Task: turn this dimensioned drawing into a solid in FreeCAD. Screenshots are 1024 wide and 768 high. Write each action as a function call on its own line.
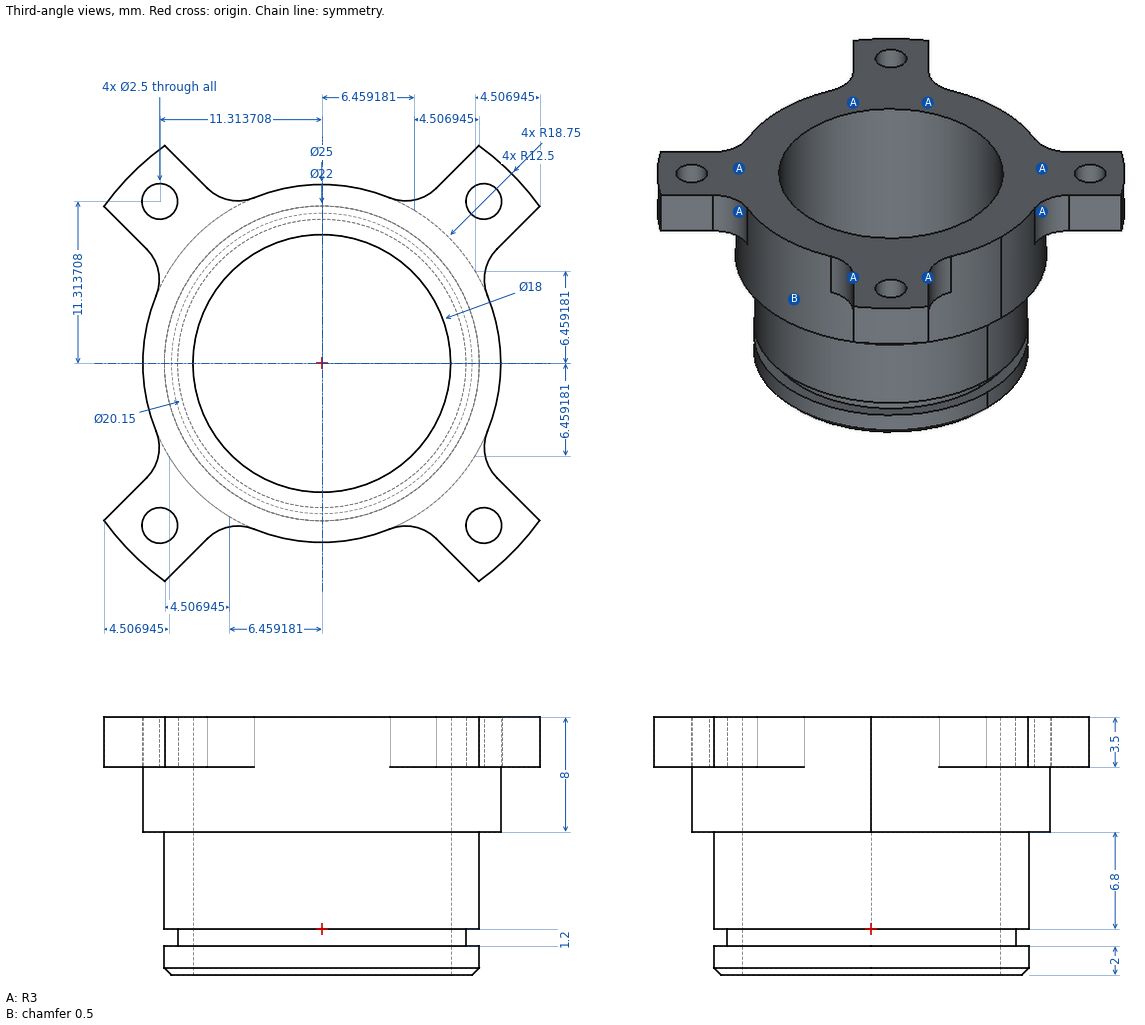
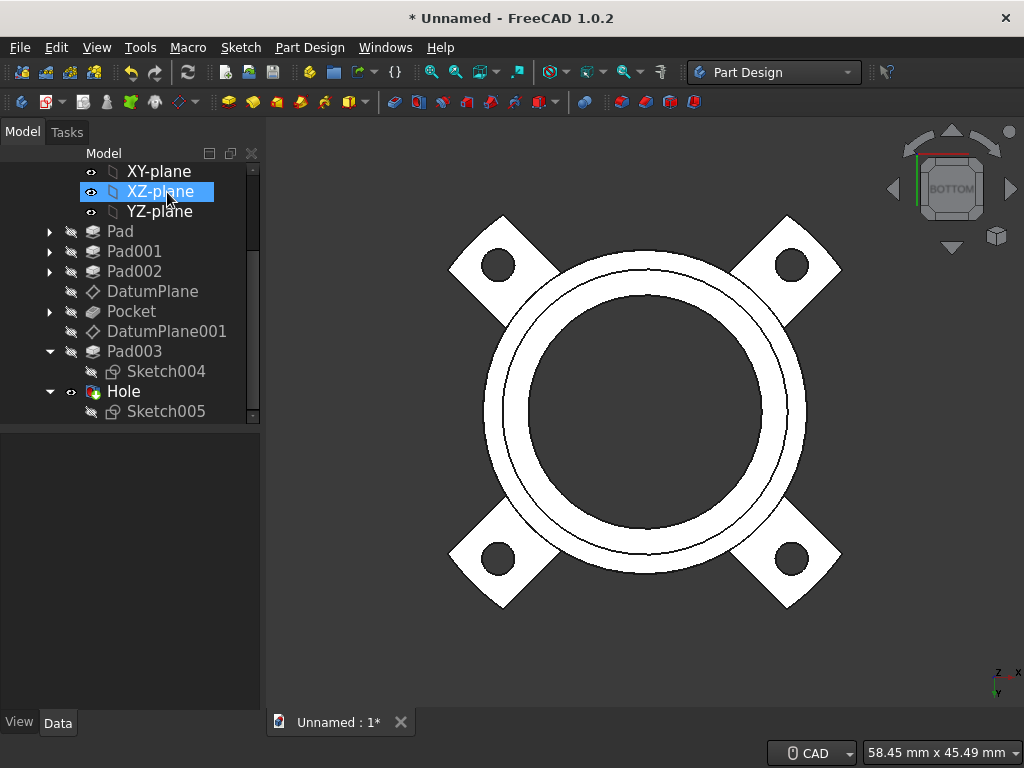
key(4)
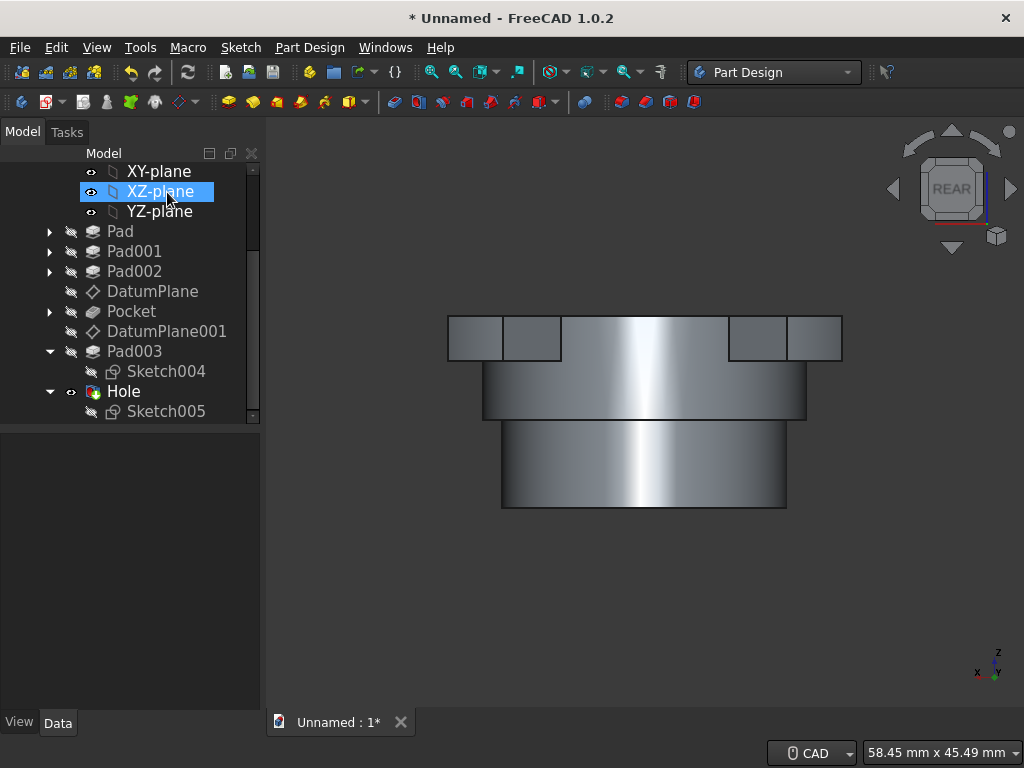
key(6)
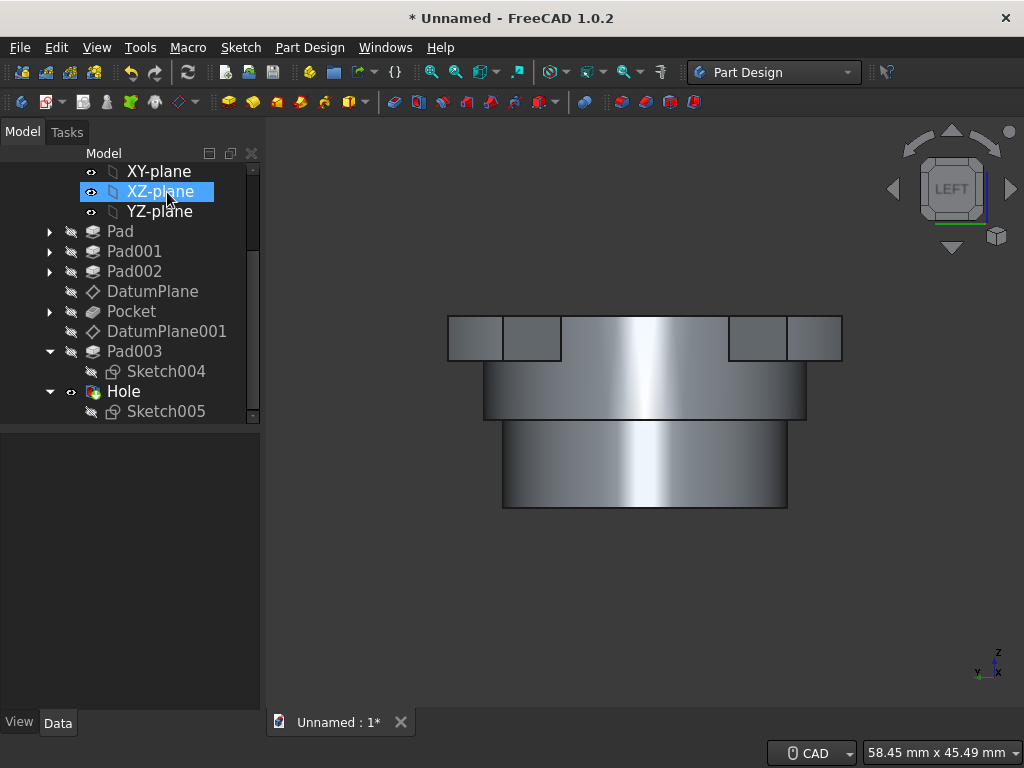
key(v)
key(3)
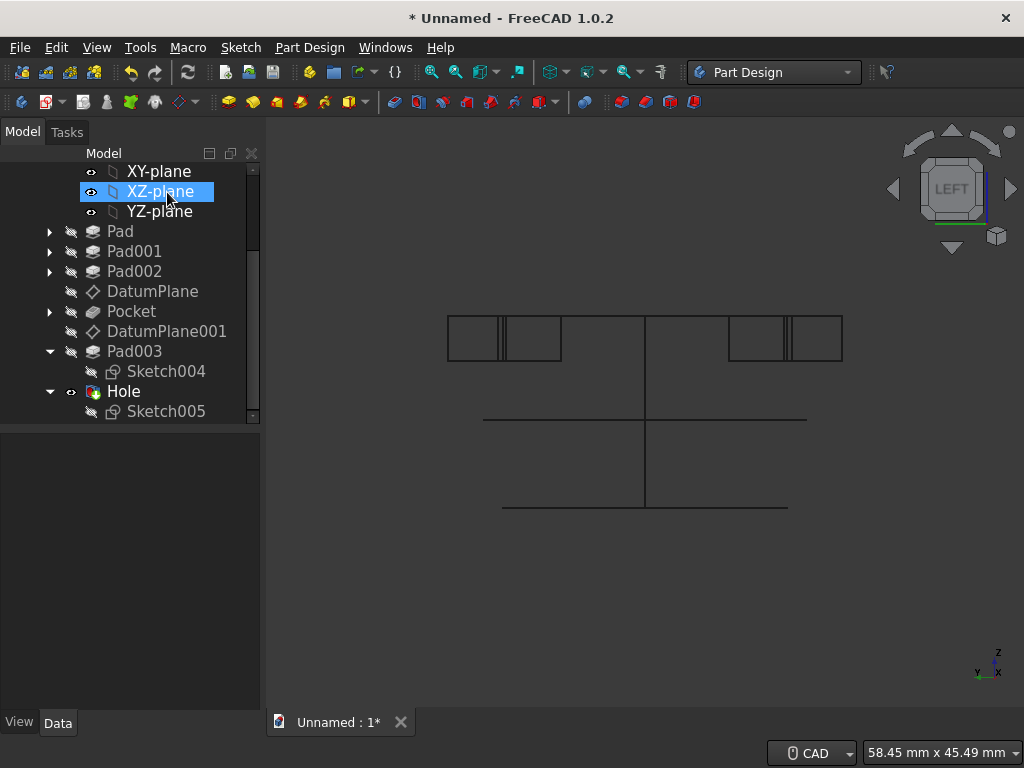
key(0)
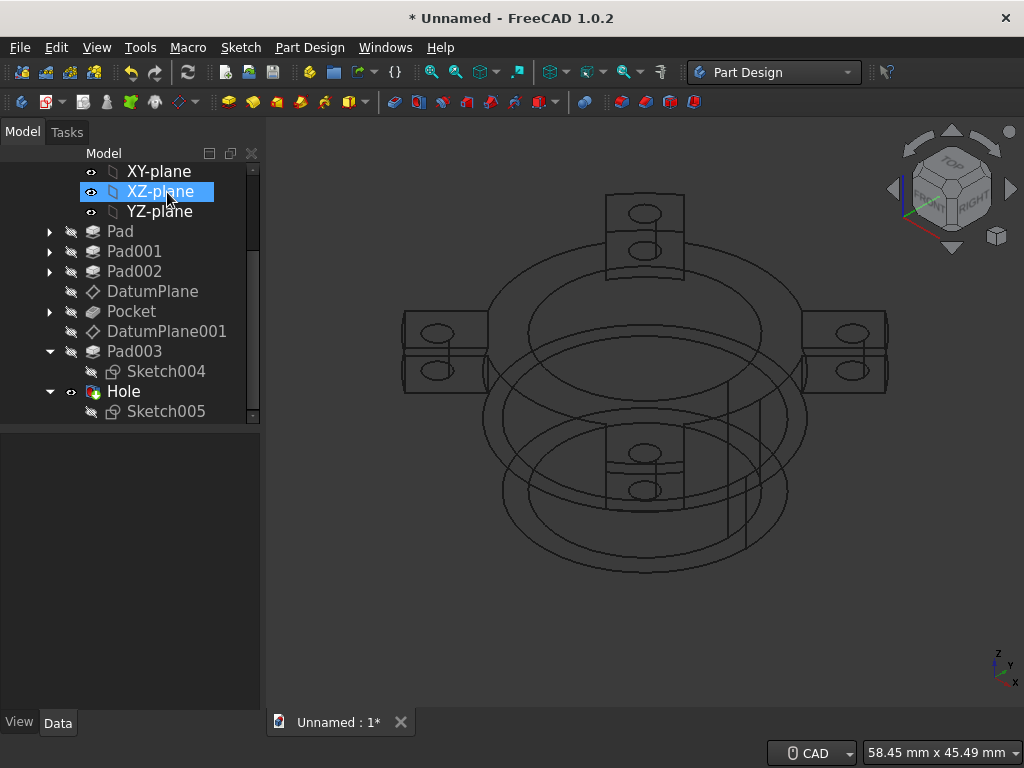
click(802, 374)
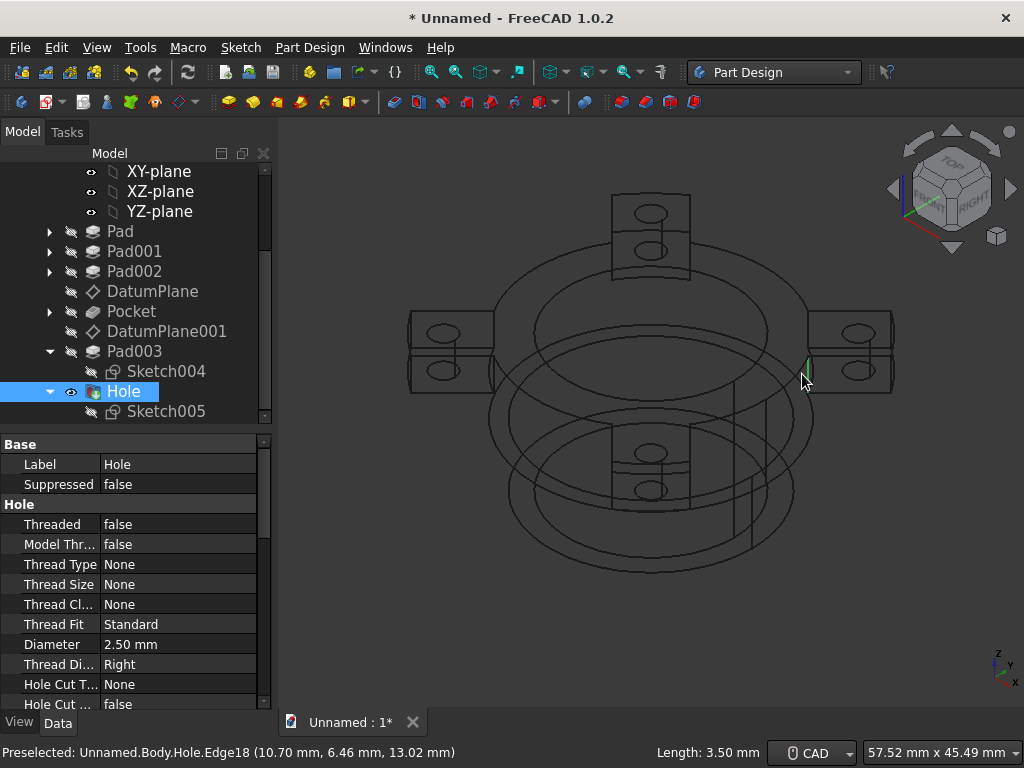
click(808, 329, ctrl)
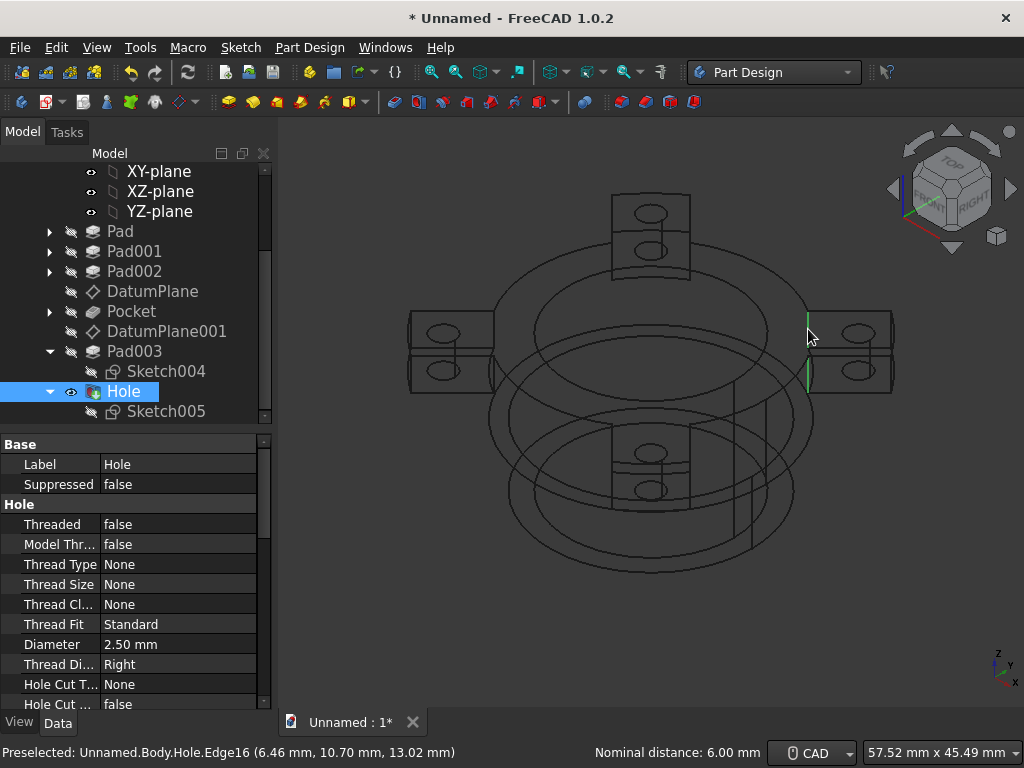
click(494, 329, ctrl)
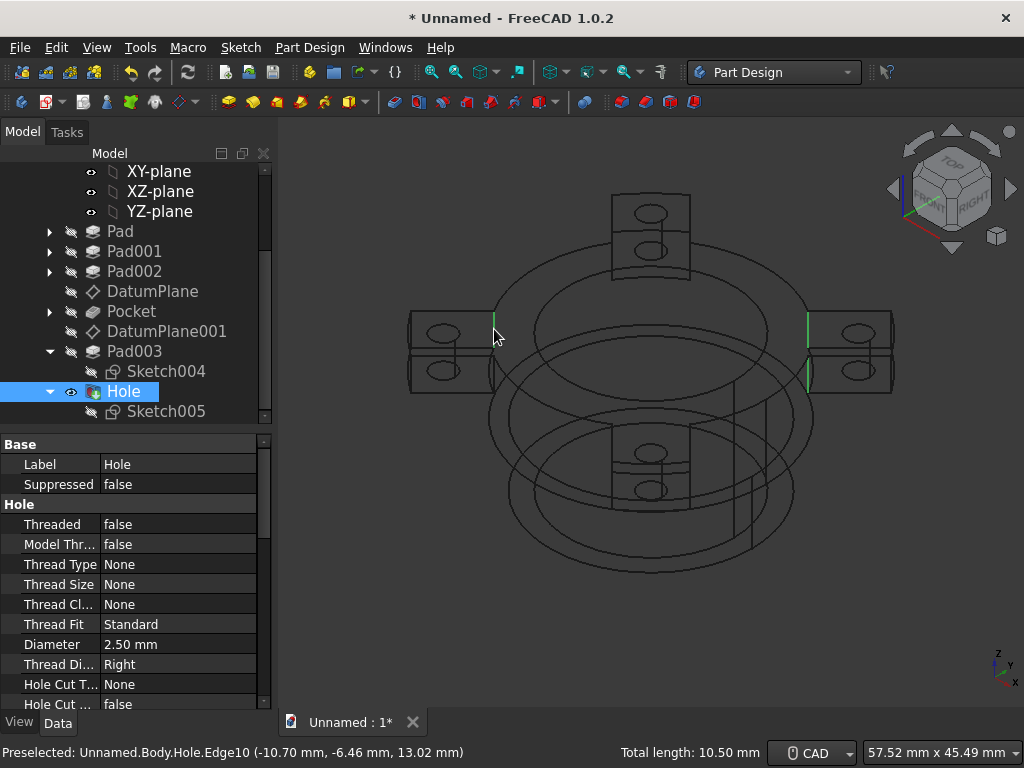
click(494, 374, ctrl)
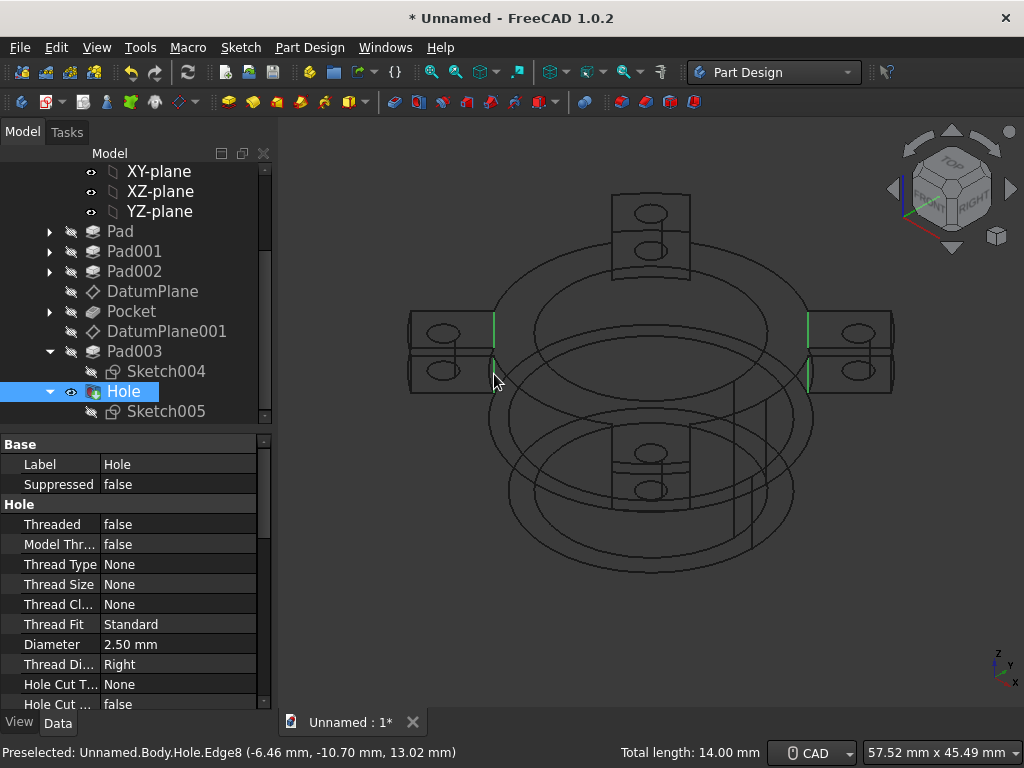
click(690, 260, ctrl)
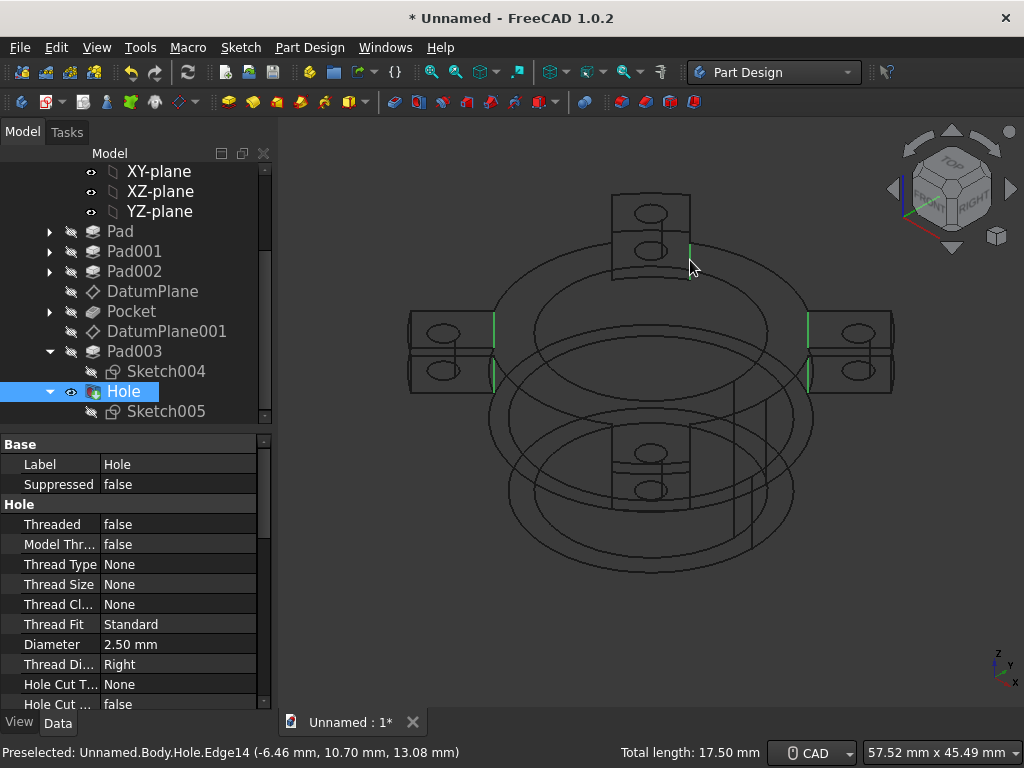
click(612, 260, ctrl)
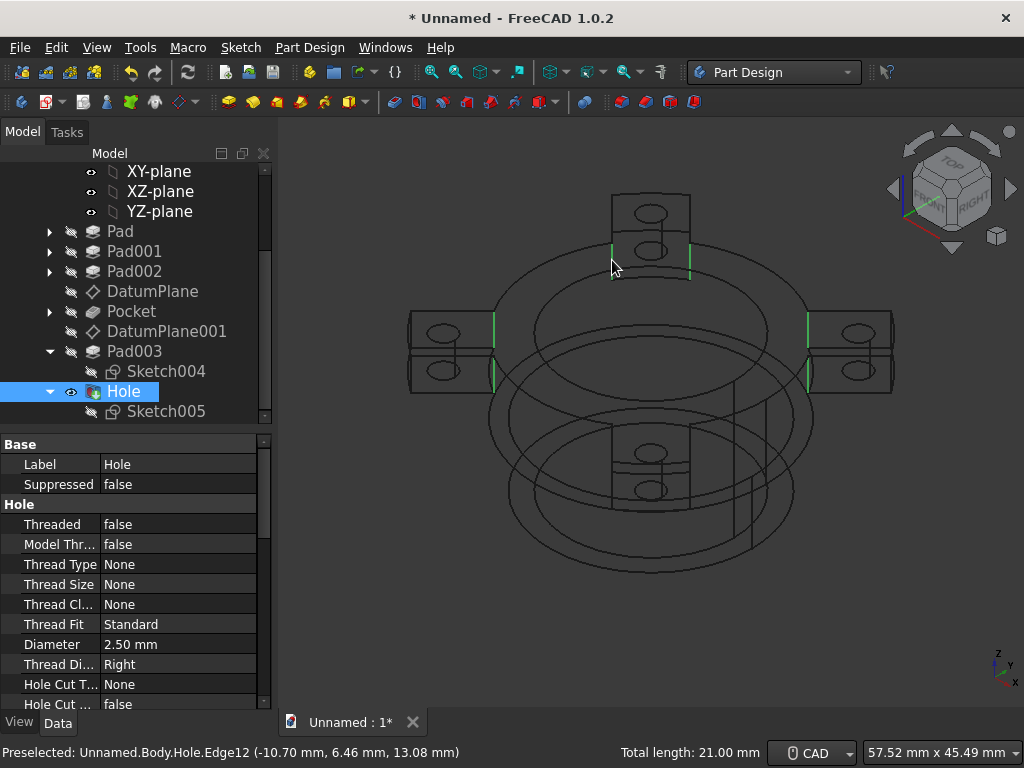
key(2)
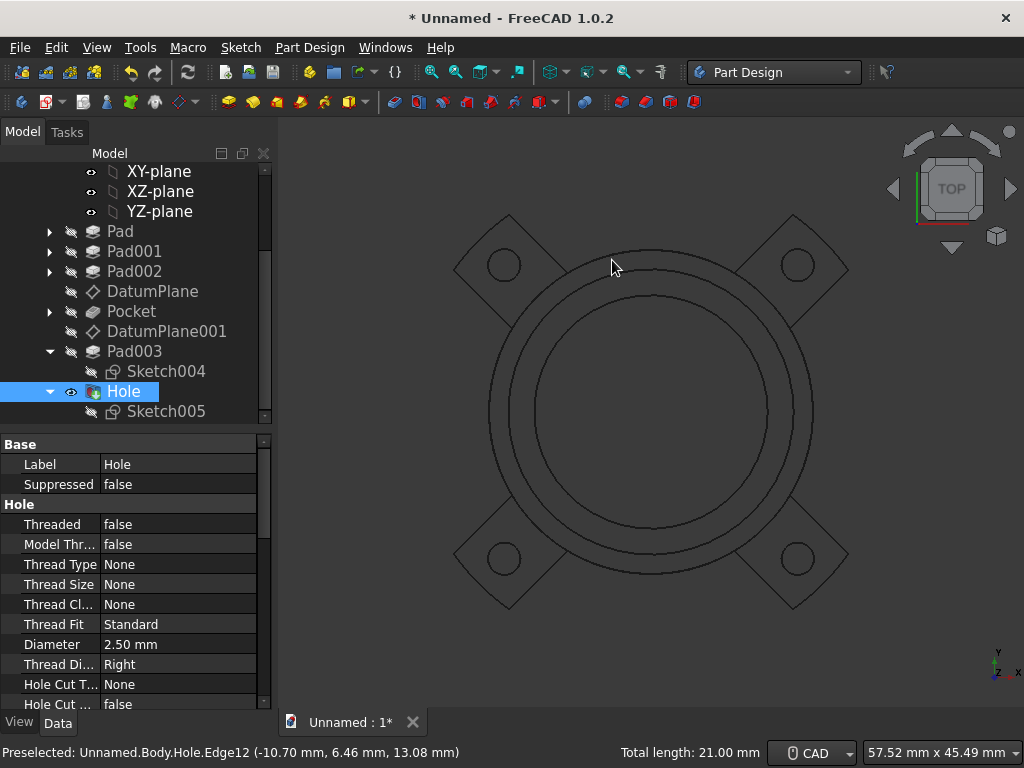
key(1)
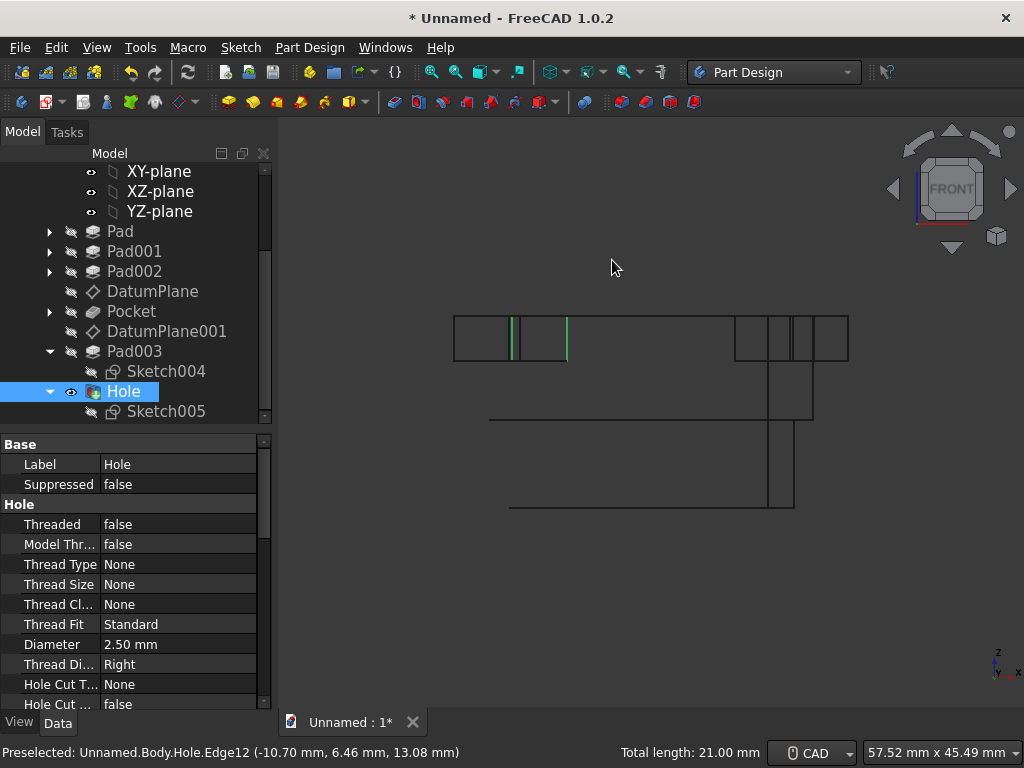
click(735, 338, ctrl)